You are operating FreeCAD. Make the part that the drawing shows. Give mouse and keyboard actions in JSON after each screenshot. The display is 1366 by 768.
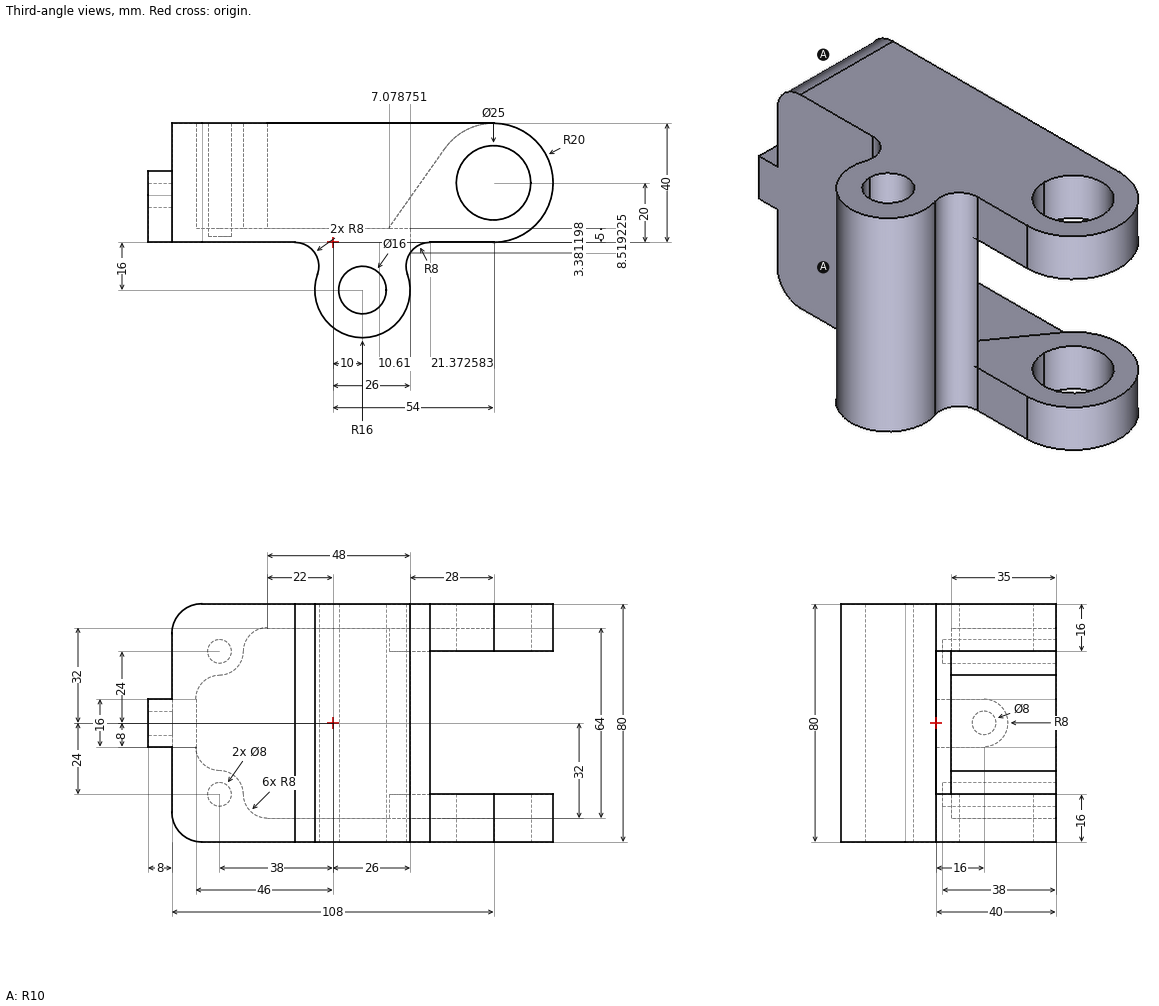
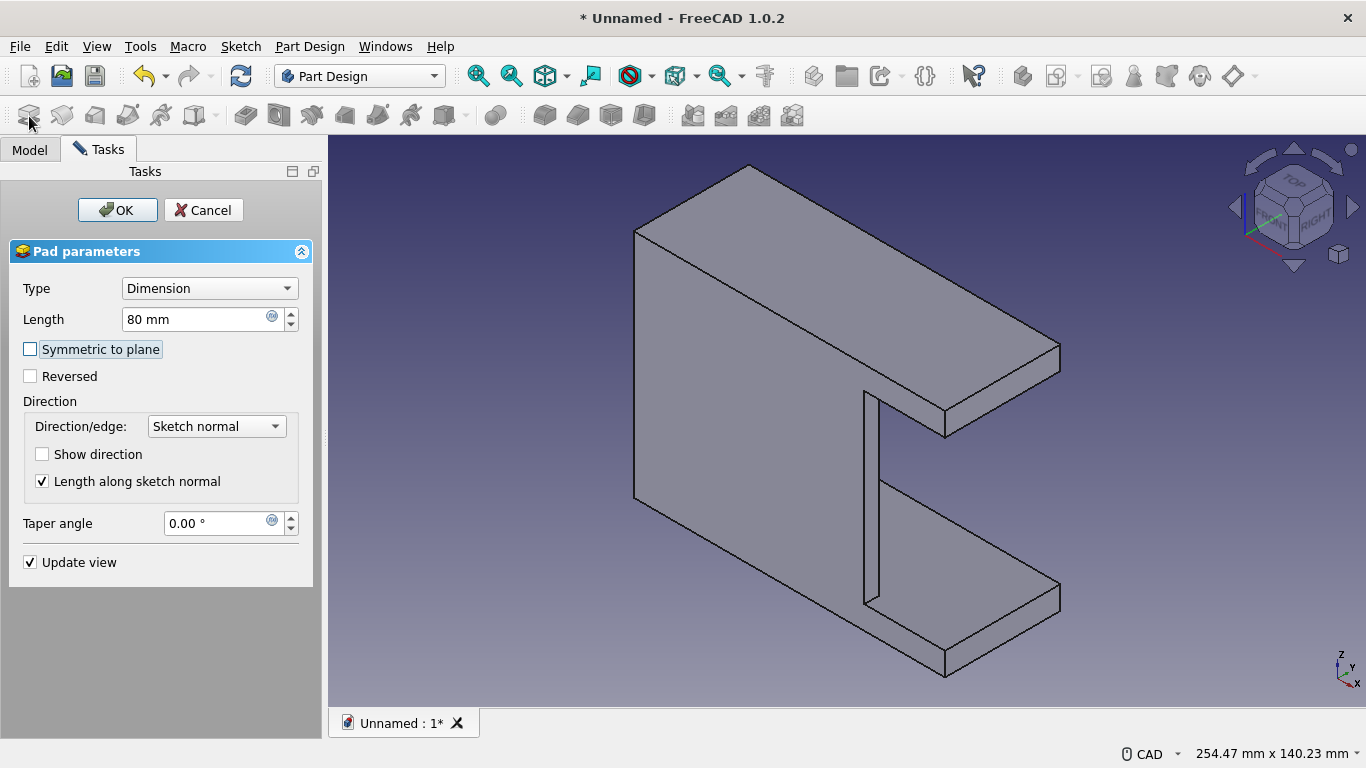
{"action": "left_click", "coordinate": [31, 376]}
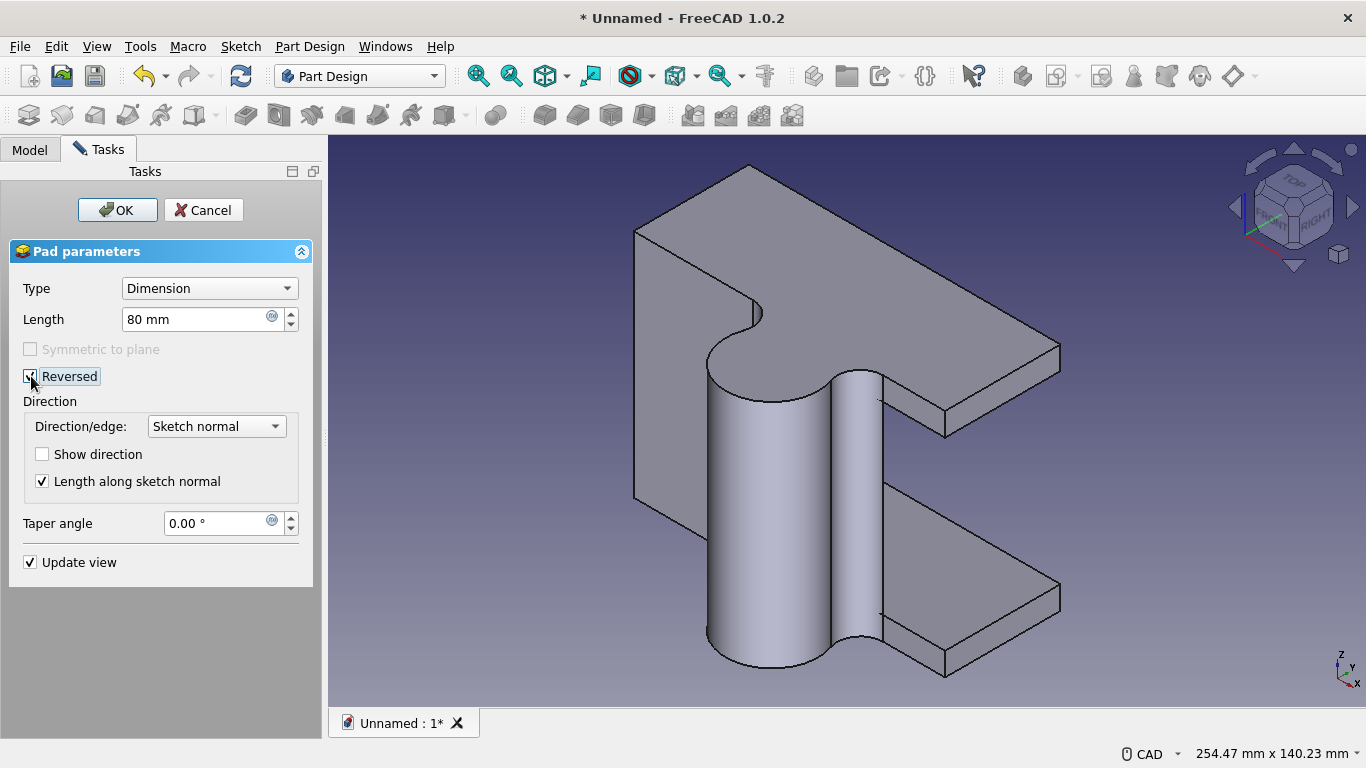
{"action": "left_click", "coordinate": [118, 210]}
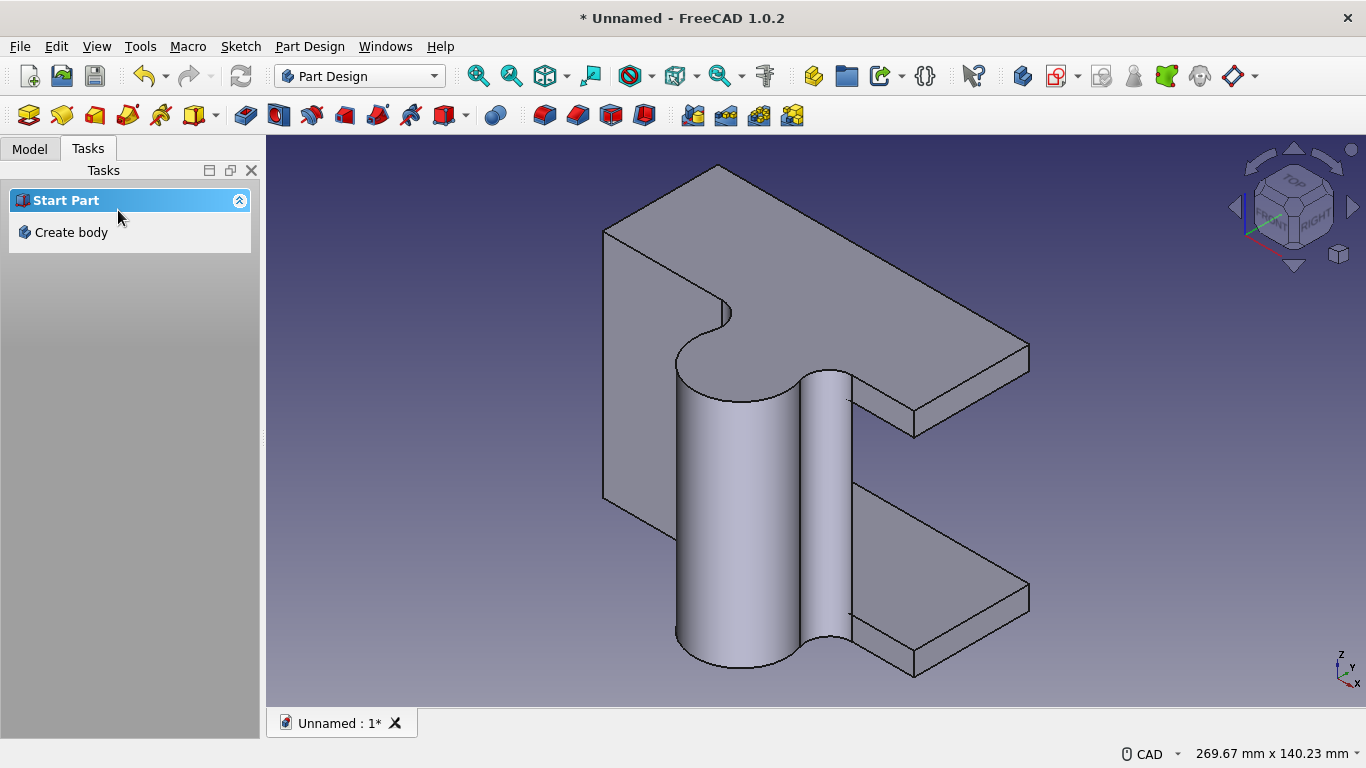
{"action": "key", "text": "v f"}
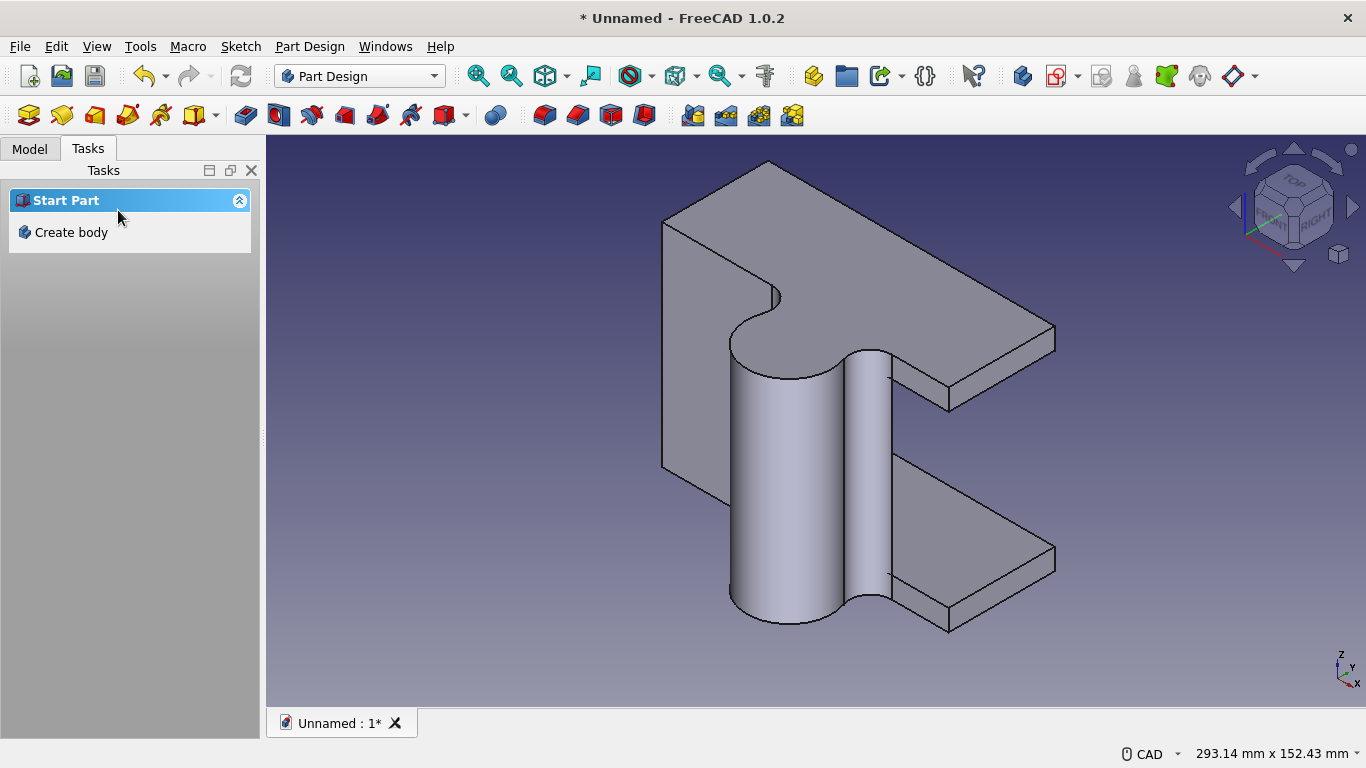
{"action": "left_click", "coordinate": [884, 305]}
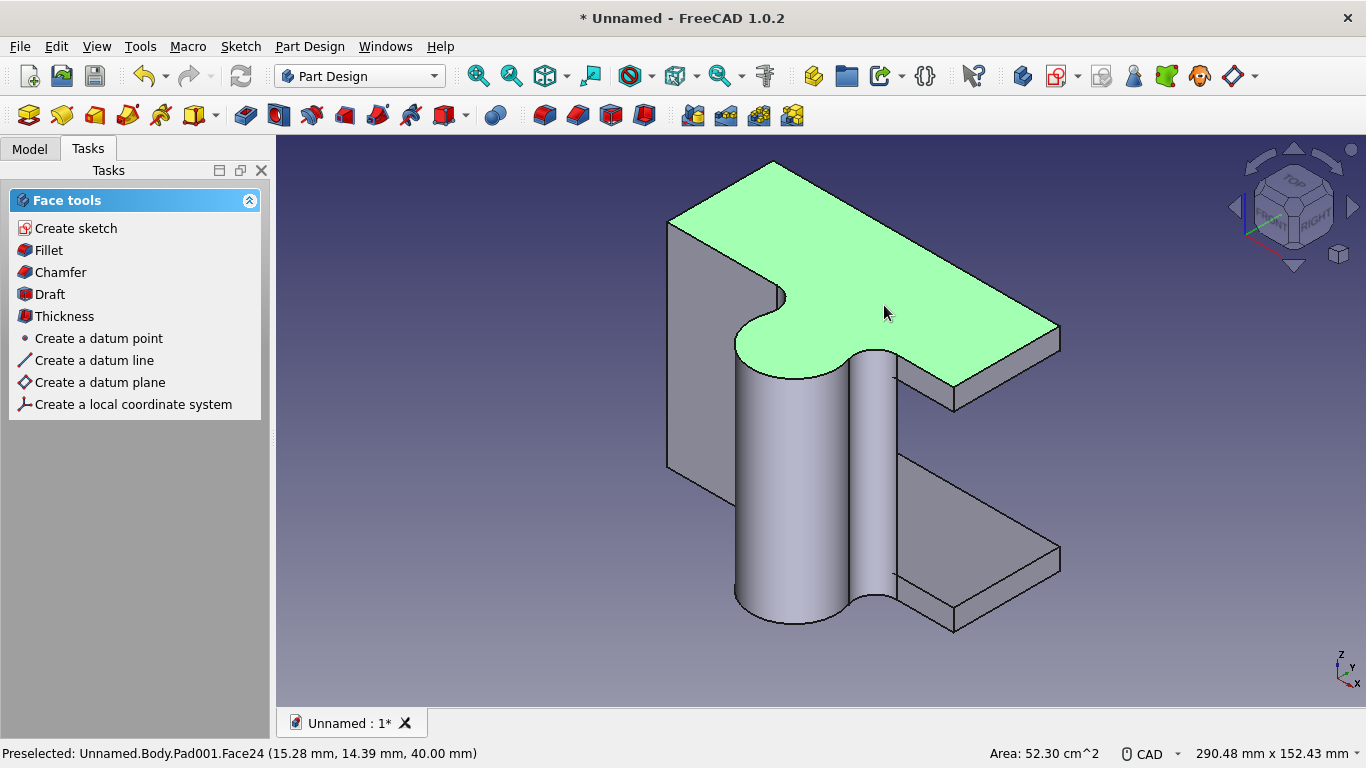
{"action": "left_click", "coordinate": [1056, 76]}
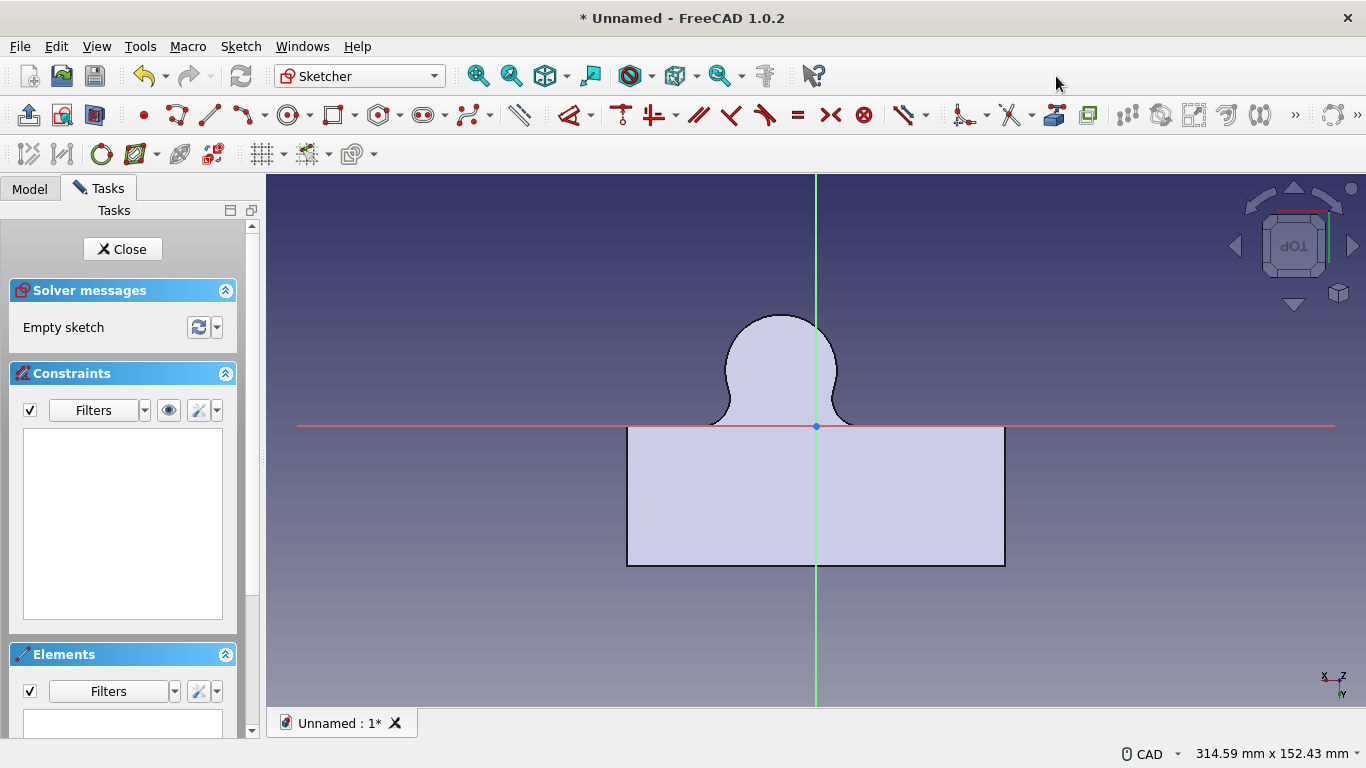
{"action": "scroll", "coordinate": [657, 496], "scroll_direction": "up", "scroll_amount": 5}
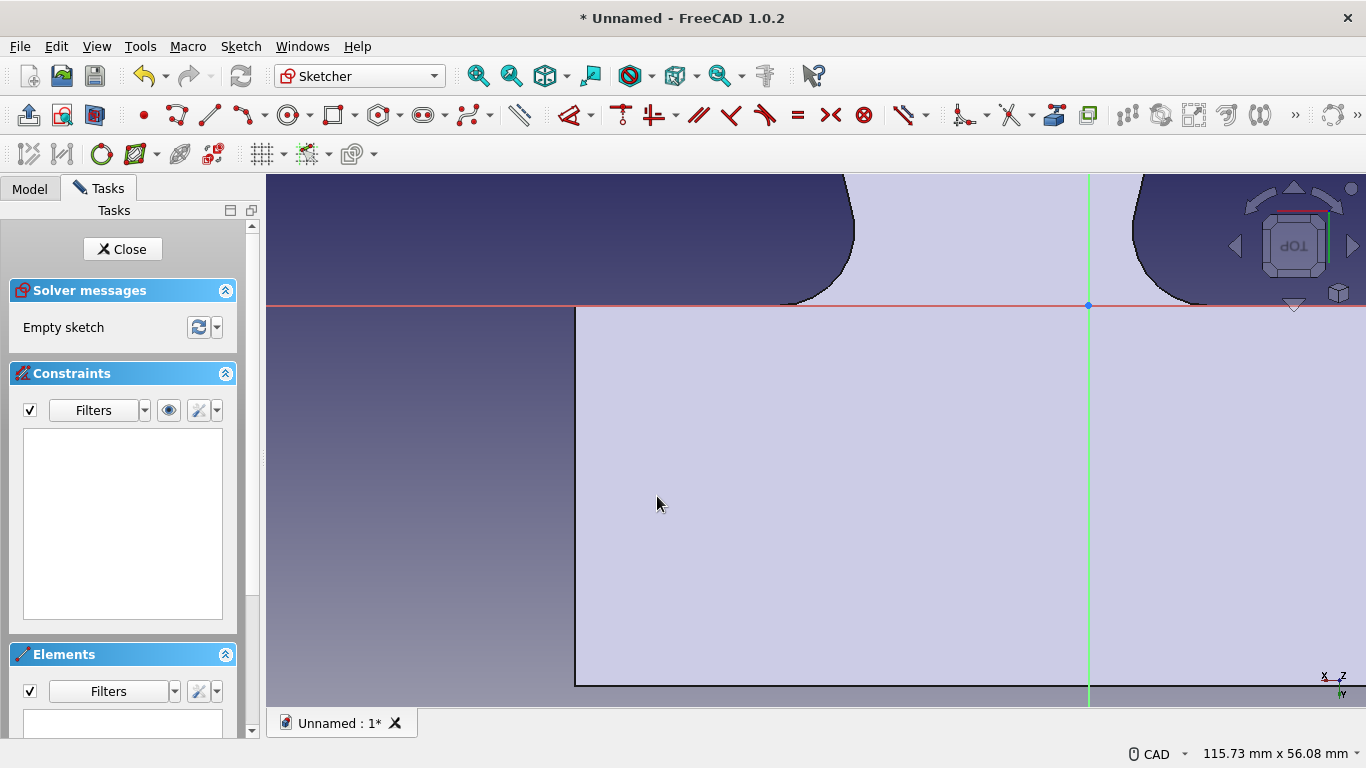
{"action": "key", "text": "g m"}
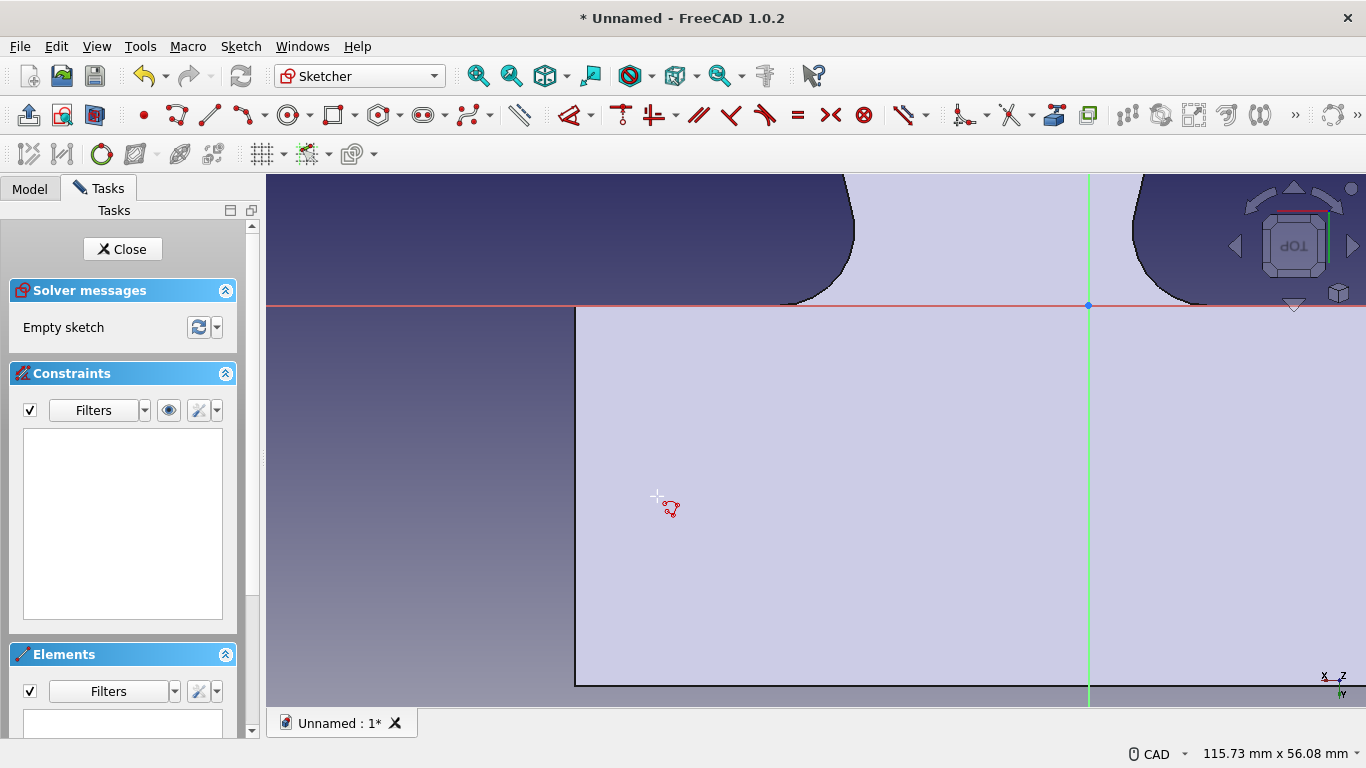
{"action": "left_click", "coordinate": [731, 605]}
{"action": "left_click", "coordinate": [942, 306]}
{"action": "left_click", "coordinate": [841, 315]}
{"action": "left_click", "coordinate": [838, 274]}
{"action": "right_click", "coordinate": [838, 274]}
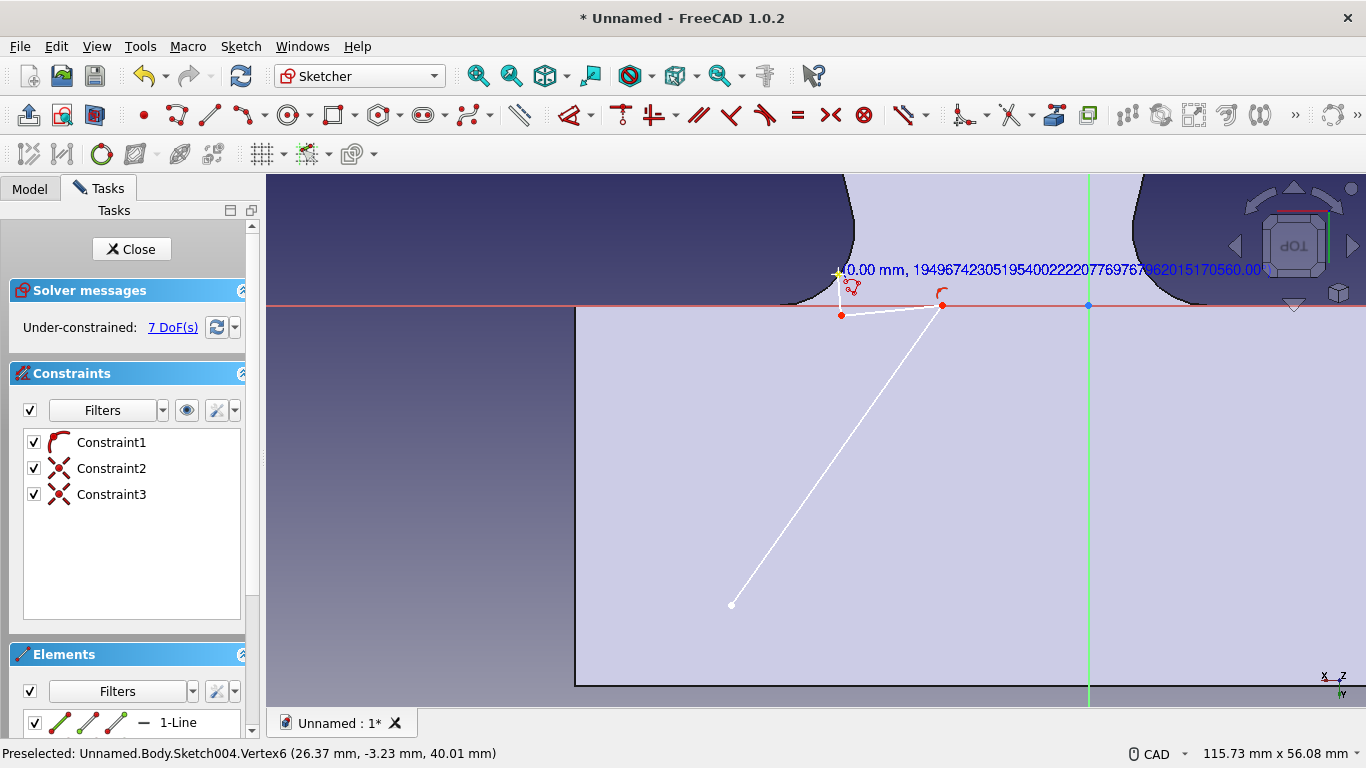
{"action": "left_click", "coordinate": [210, 116]}